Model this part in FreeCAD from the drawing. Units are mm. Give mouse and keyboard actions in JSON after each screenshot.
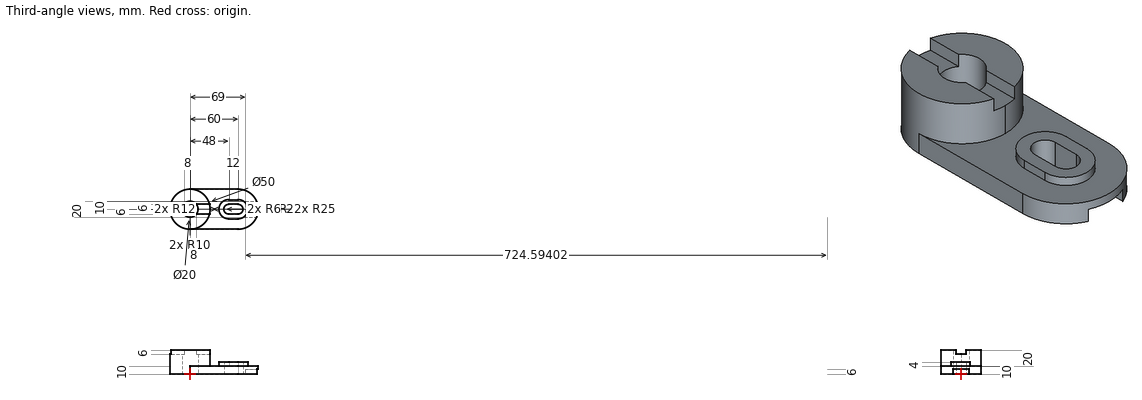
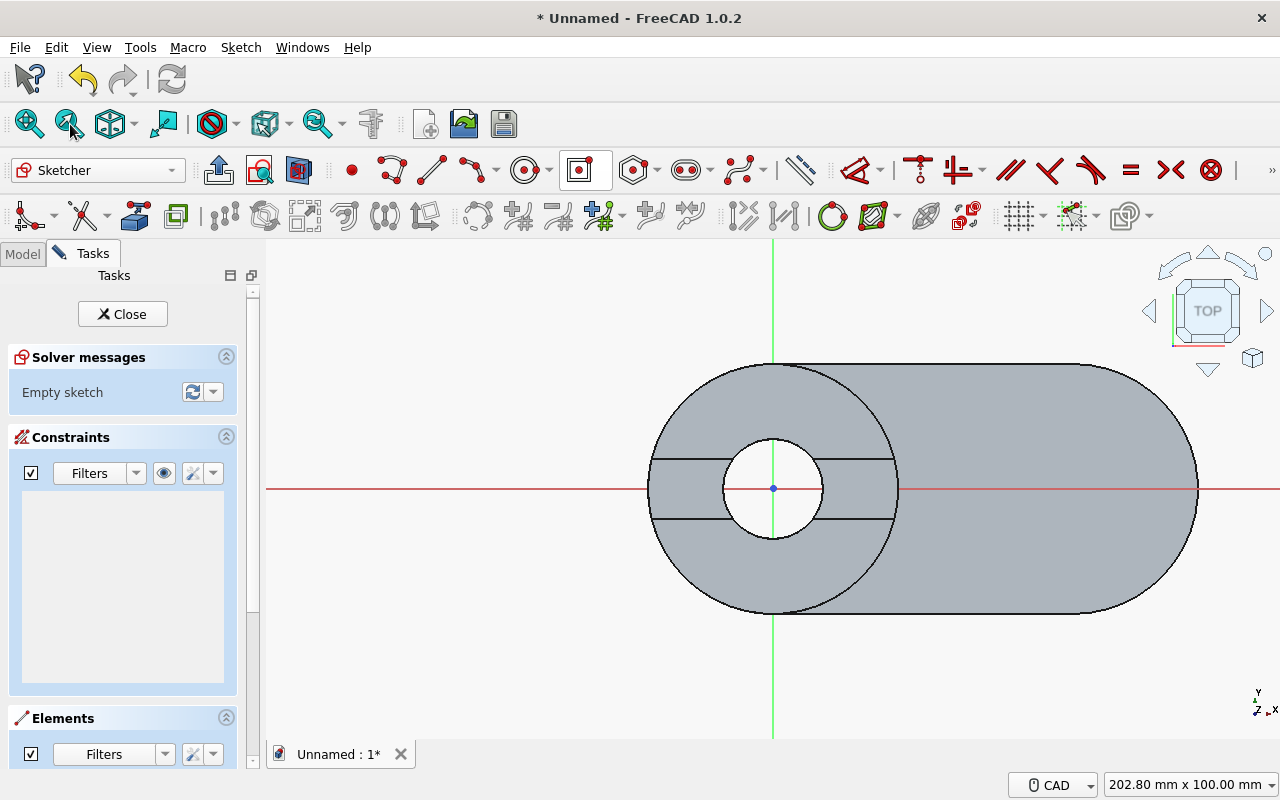
{"action": "scroll", "coordinate": [294, 489], "scroll_direction": "down", "scroll_amount": 1}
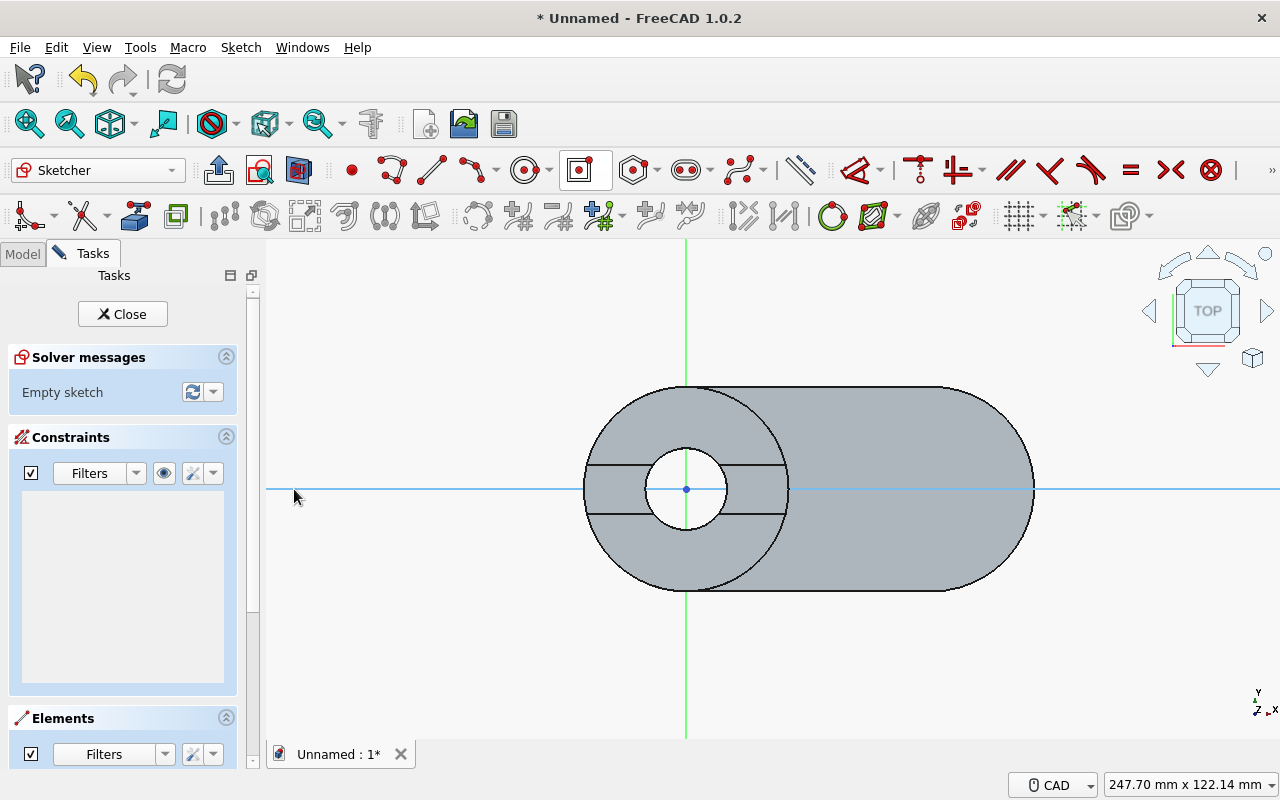
{"action": "scroll", "coordinate": [991, 489], "scroll_direction": "up", "scroll_amount": 3}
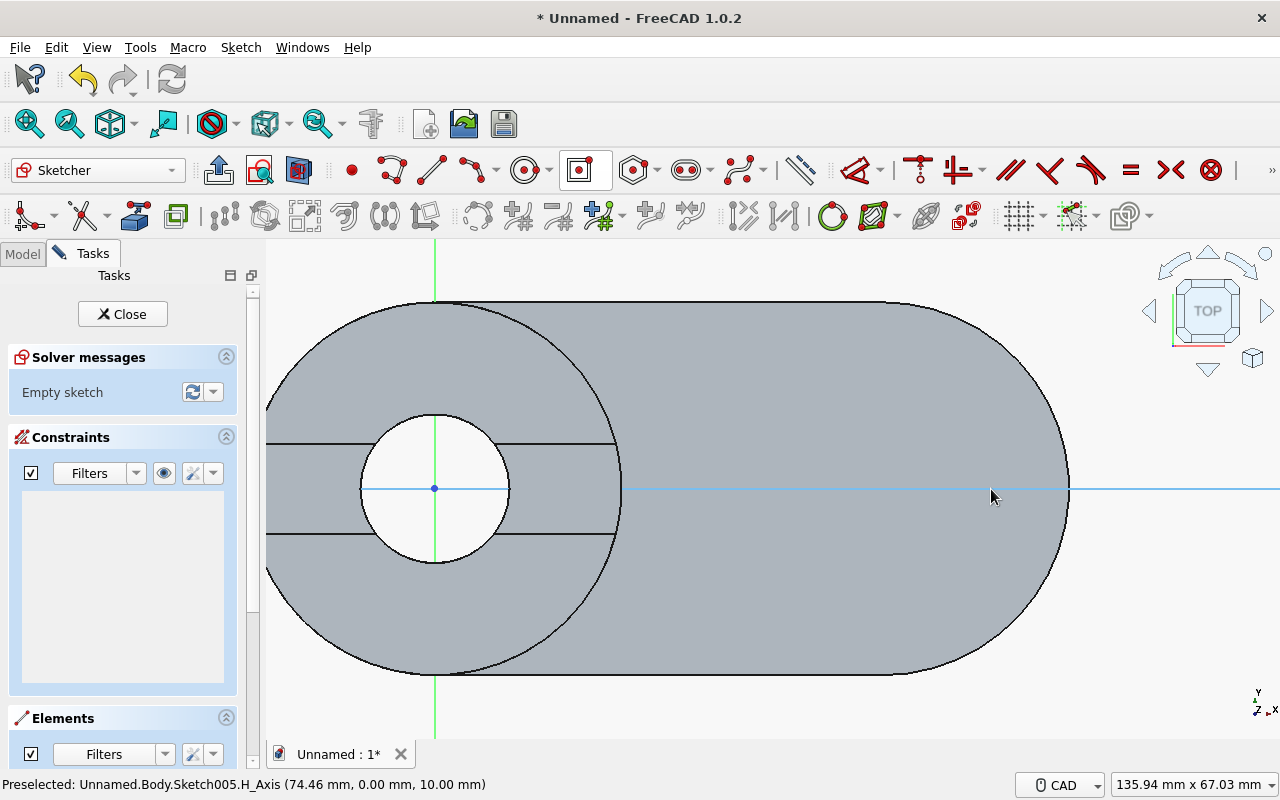
{"action": "left_click", "coordinate": [686, 170]}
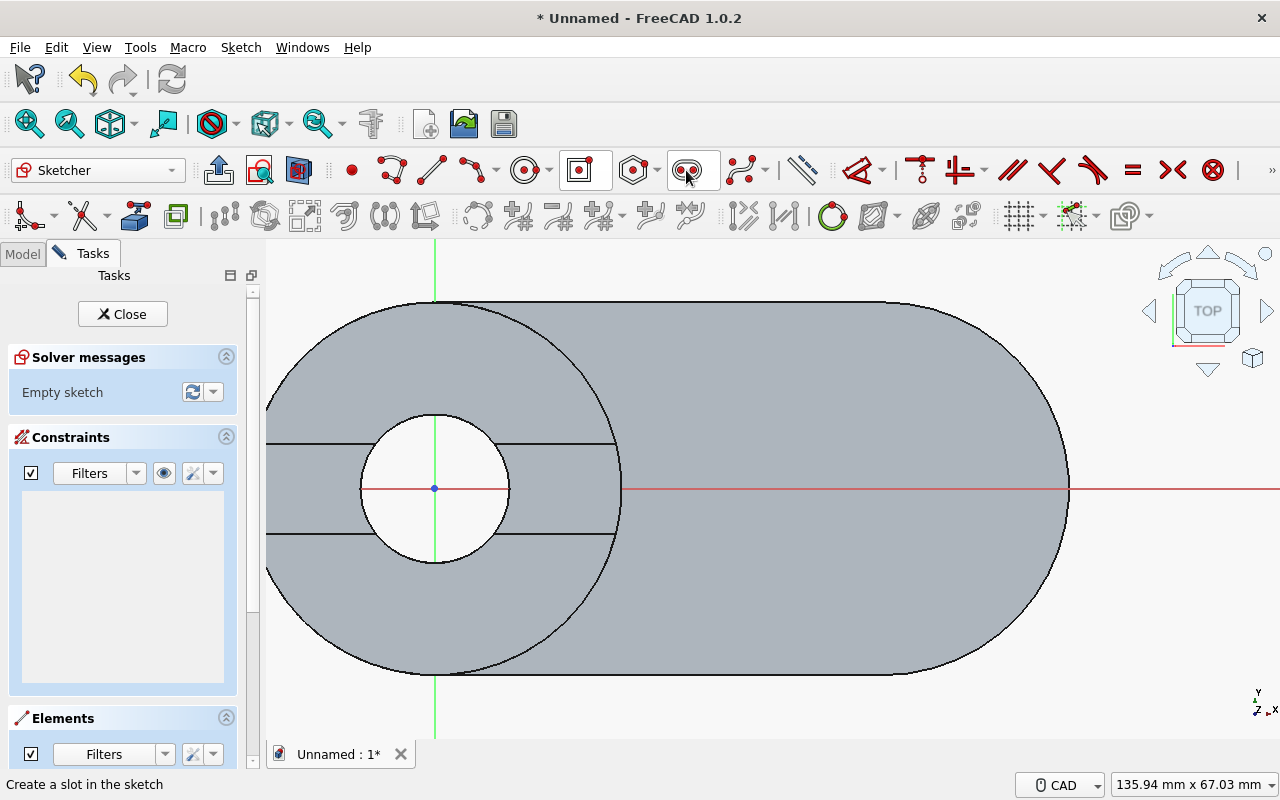
{"action": "left_click", "coordinate": [793, 489]}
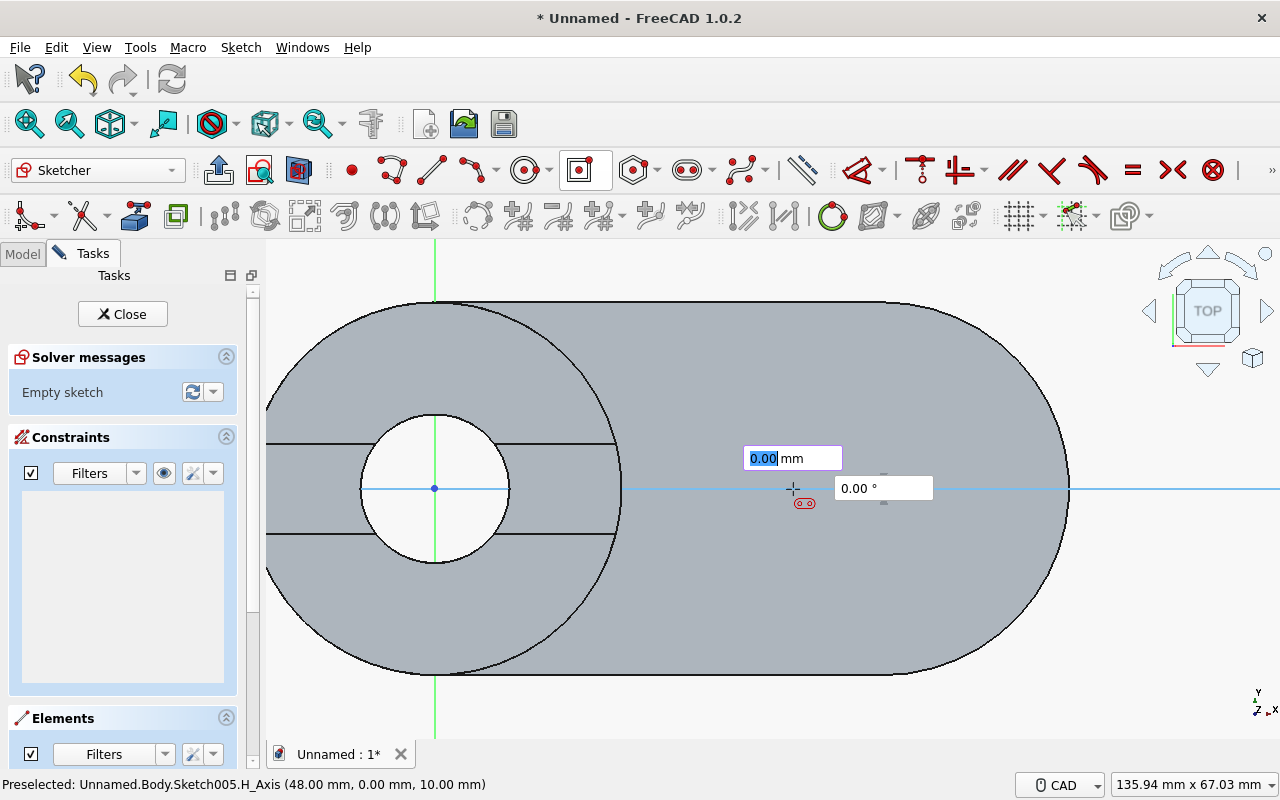
{"action": "left_click", "coordinate": [883, 480]}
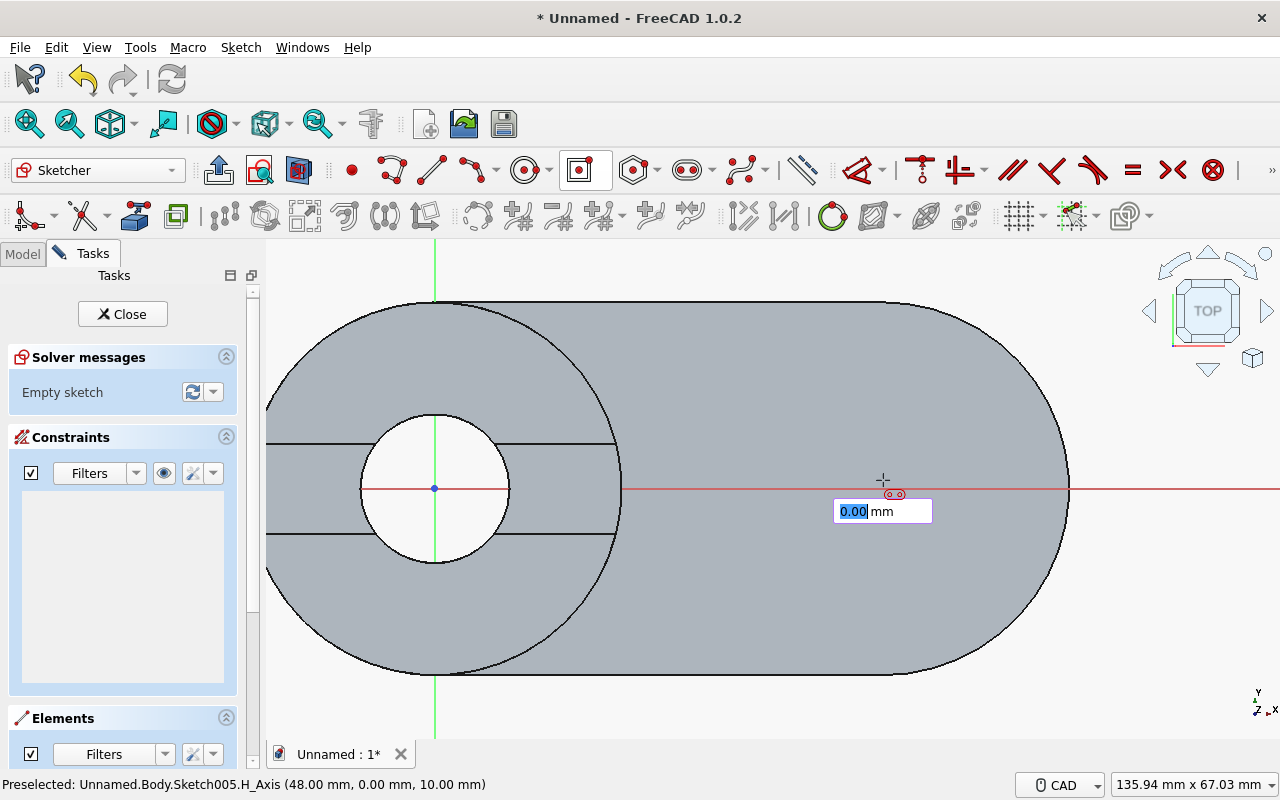
{"action": "left_click", "coordinate": [838, 399]}
{"action": "key", "text": "Escape"}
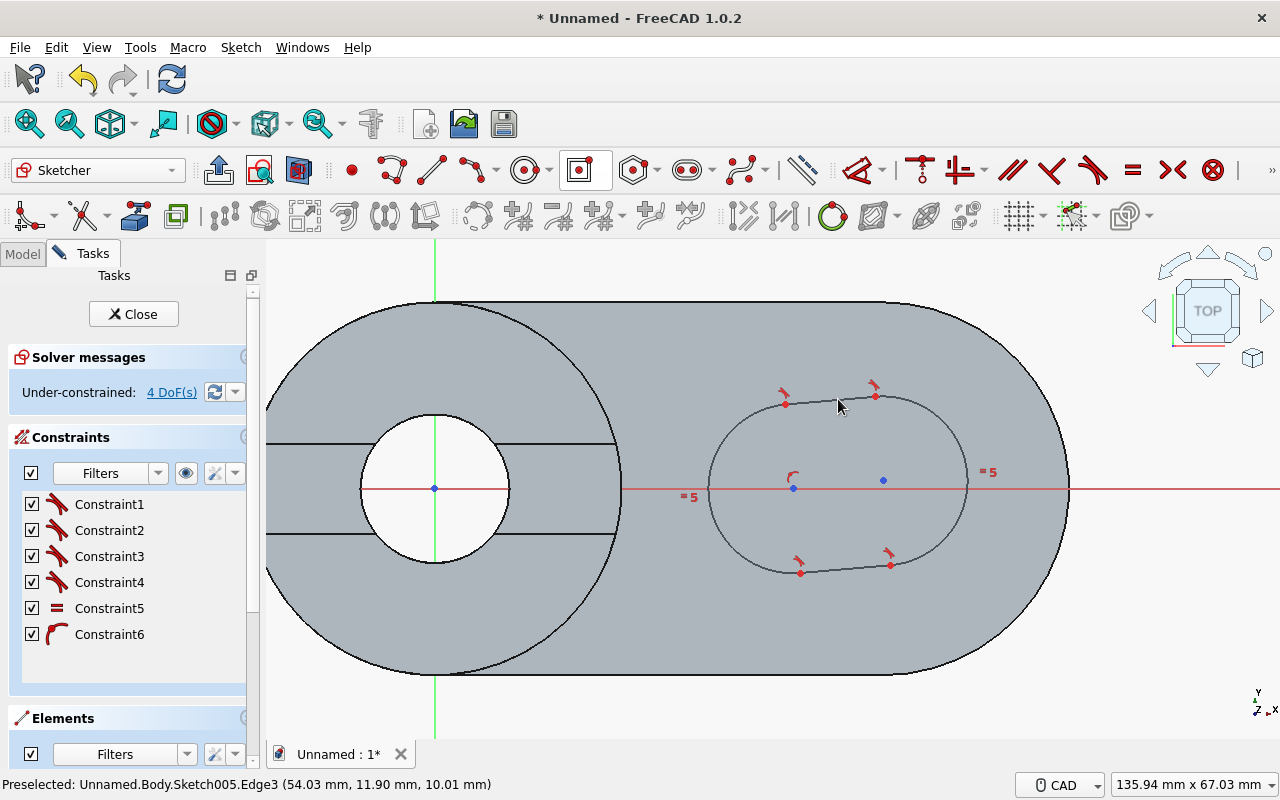
{"action": "left_click", "coordinate": [813, 402]}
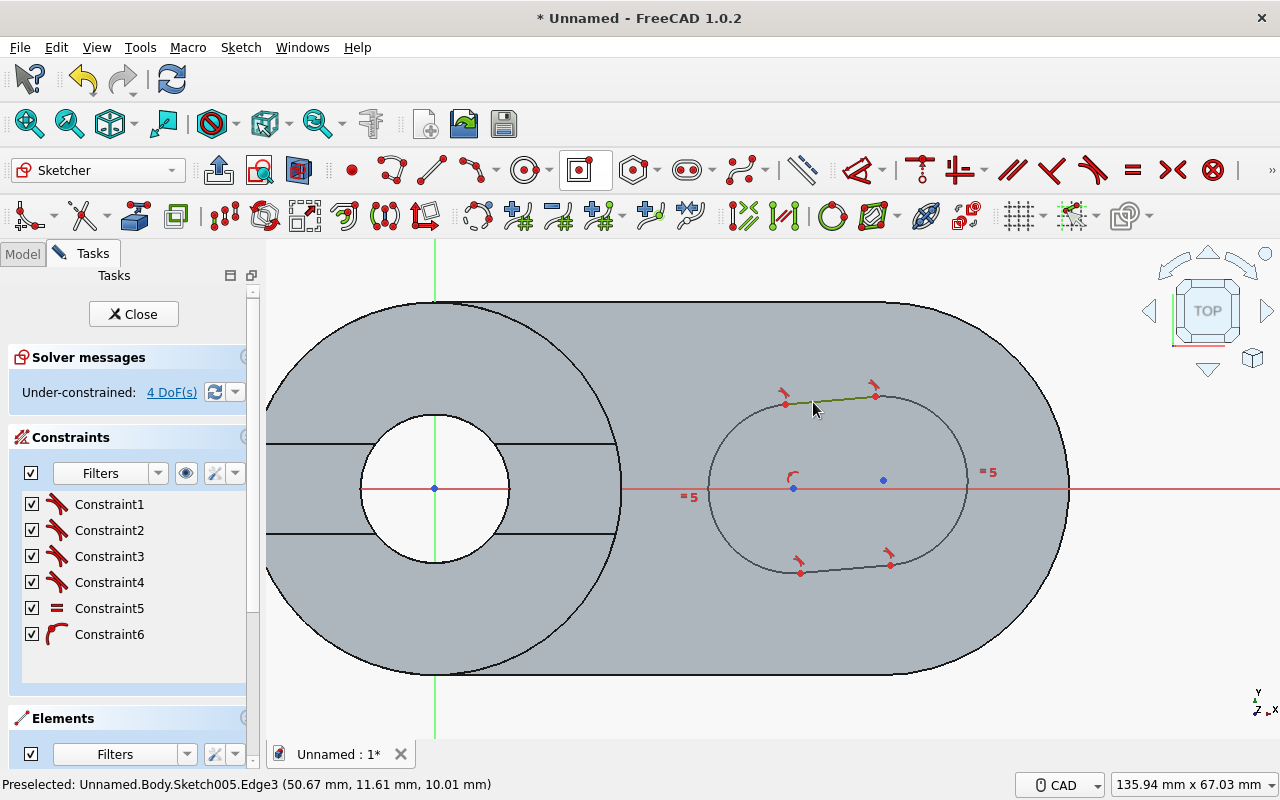
{"action": "key", "text": "h"}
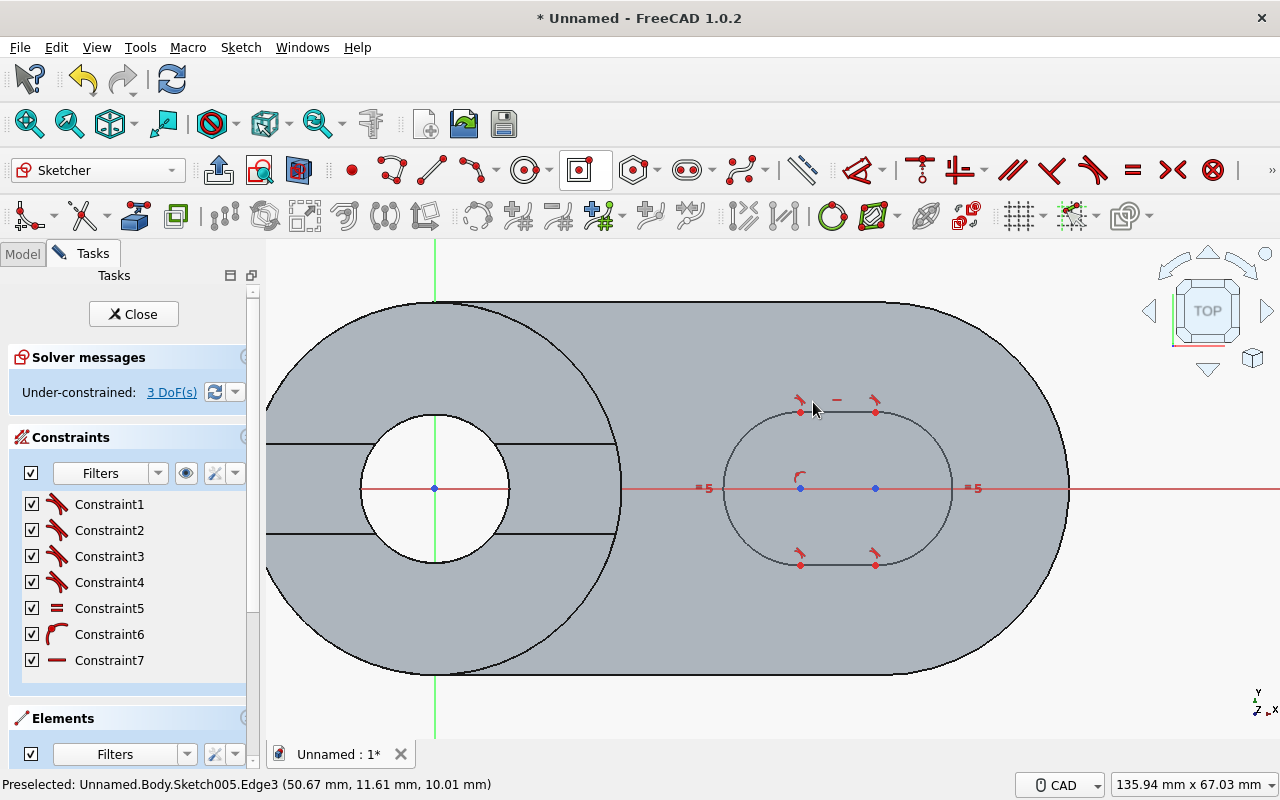
{"action": "left_click", "coordinate": [858, 170]}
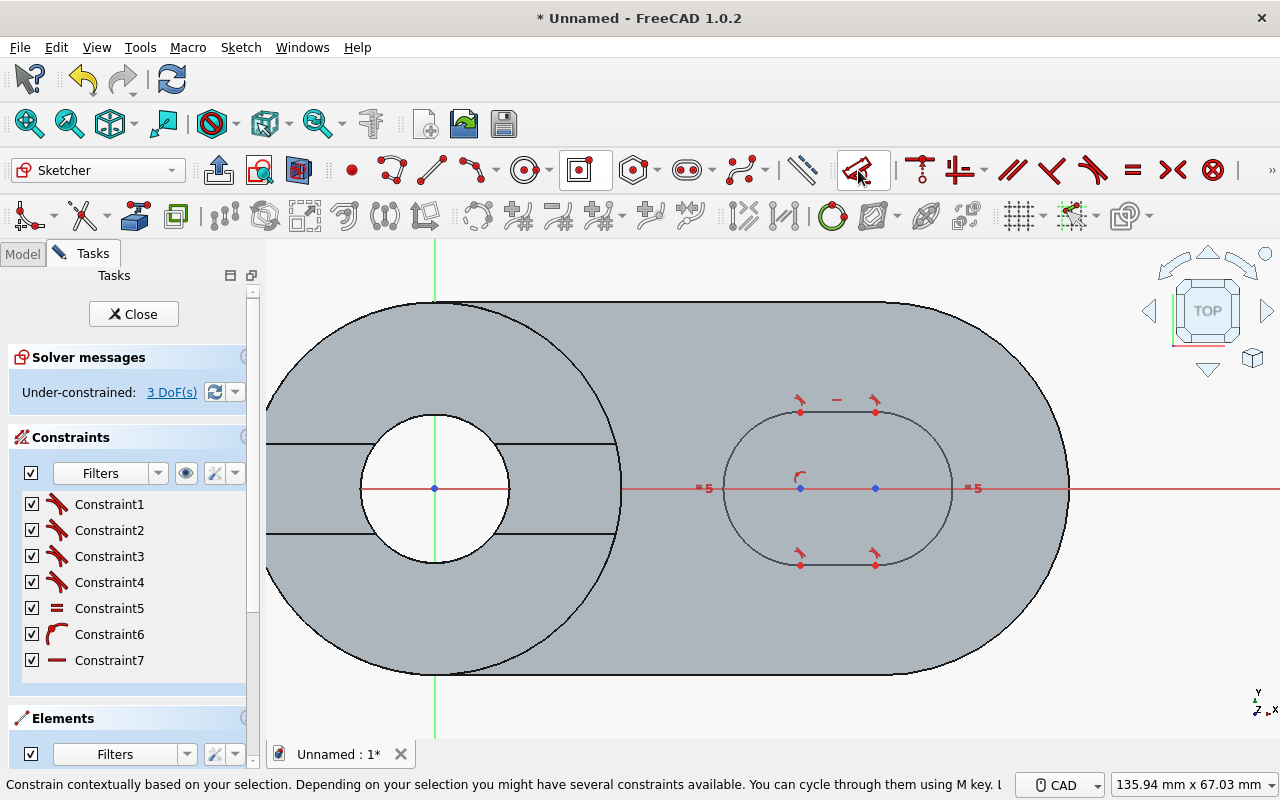
{"action": "left_click", "coordinate": [738, 444]}
{"action": "left_click", "coordinate": [712, 425]}